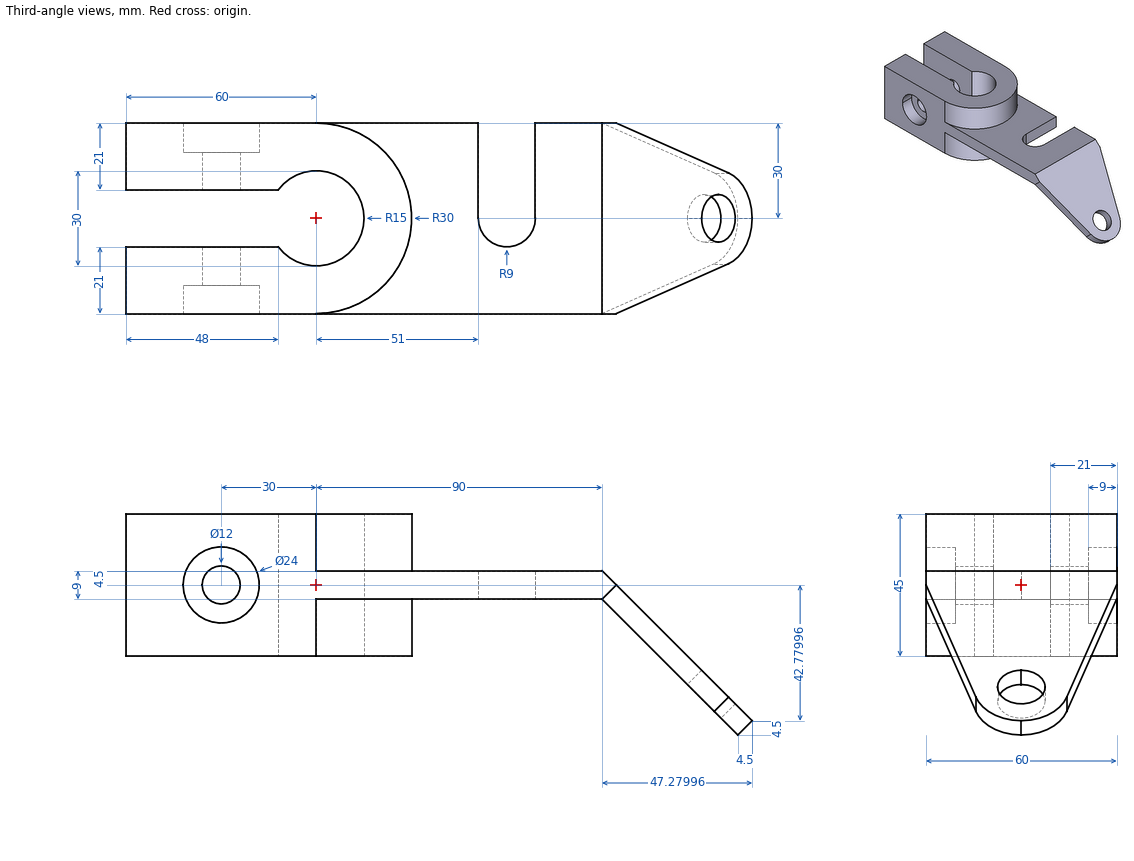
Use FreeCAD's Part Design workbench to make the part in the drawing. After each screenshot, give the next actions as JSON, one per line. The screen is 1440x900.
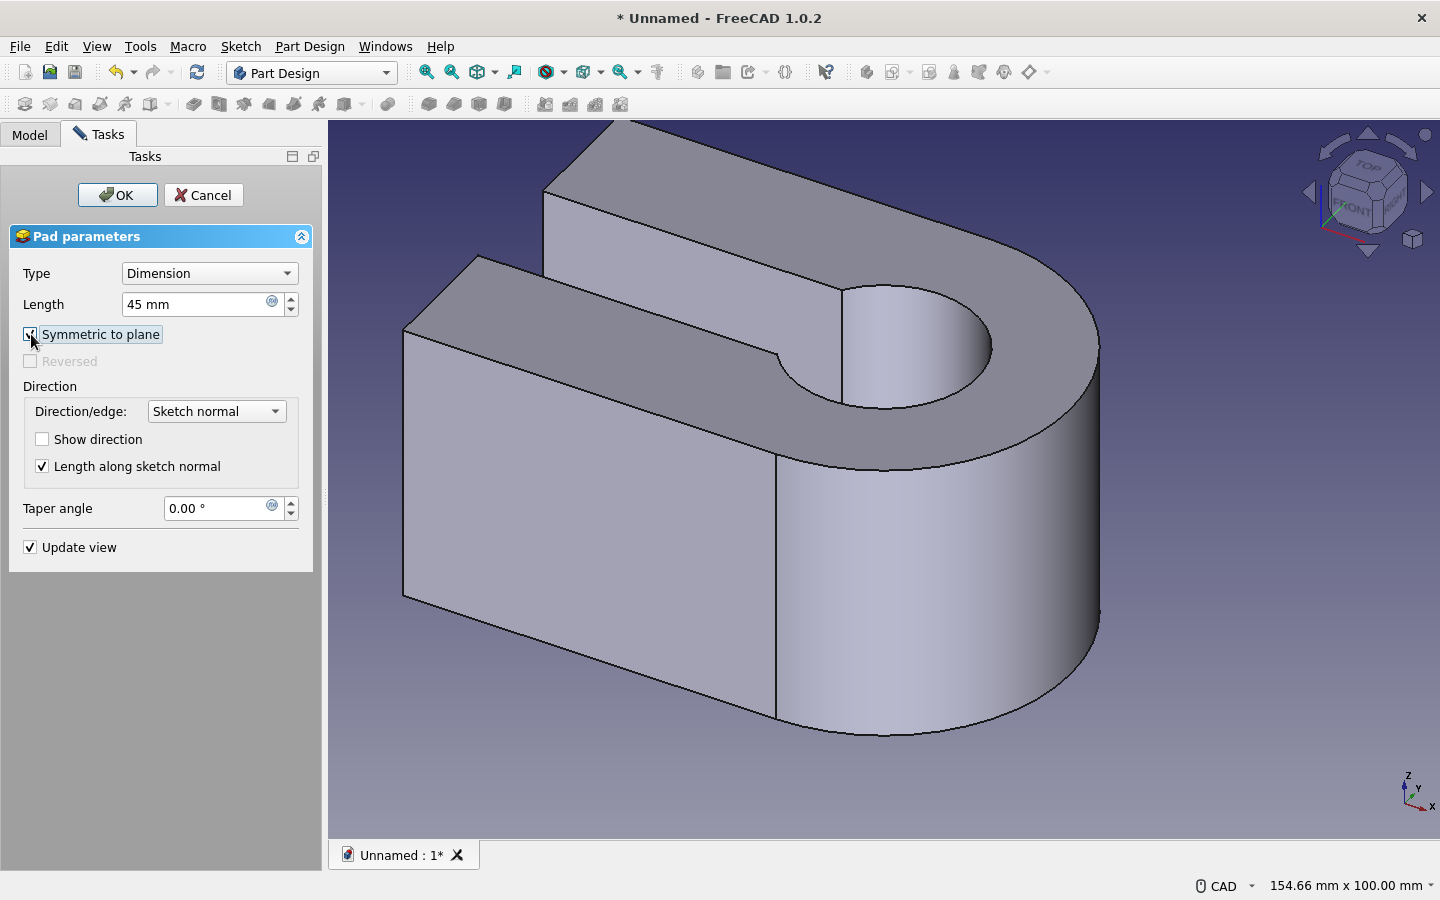
{"action": "left_click", "coordinate": [118, 195]}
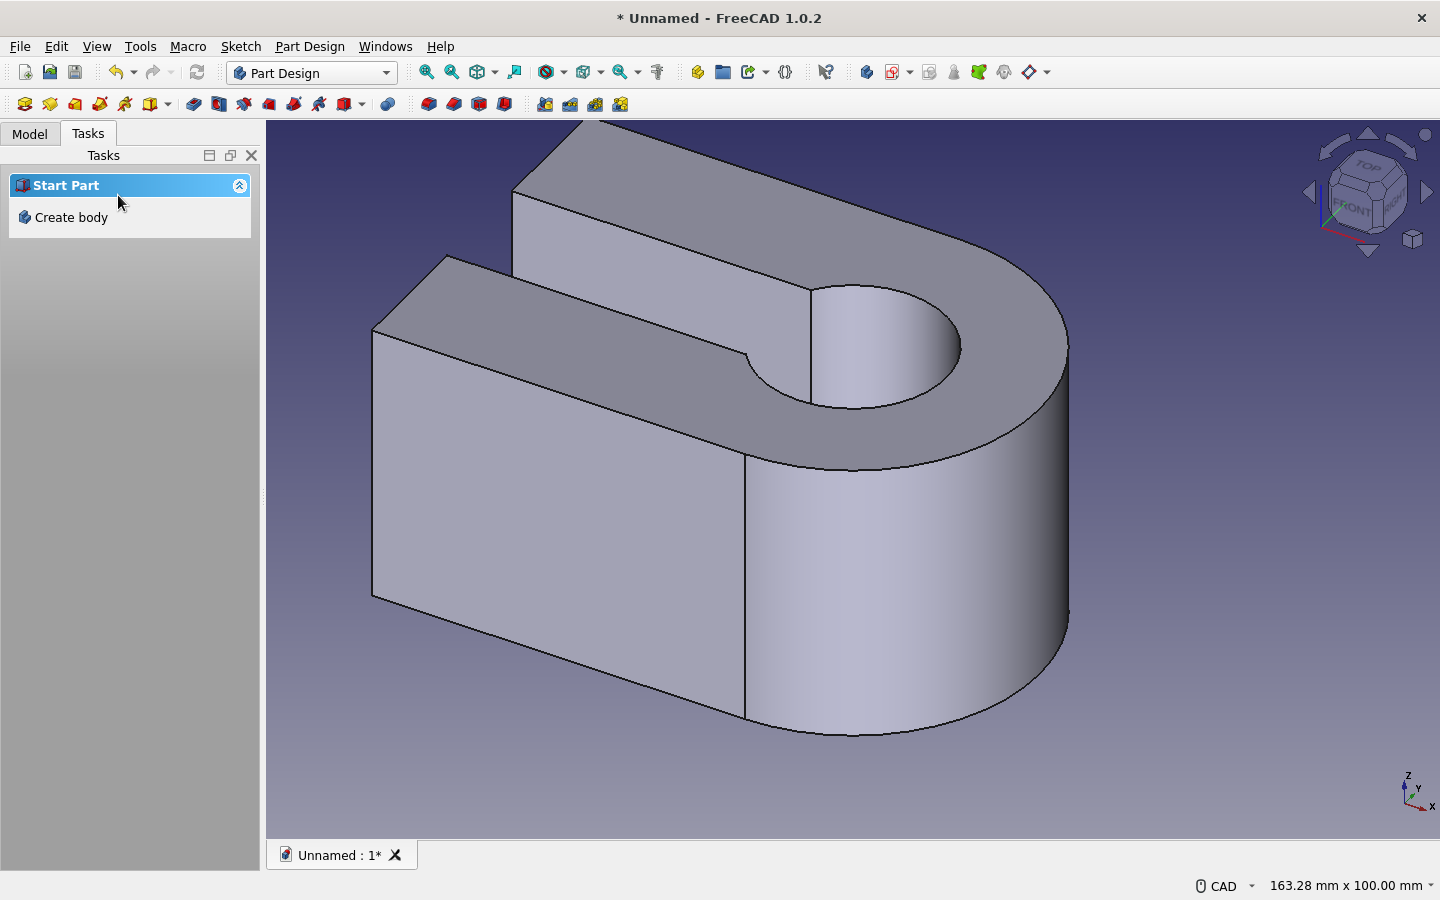
{"action": "left_click", "coordinate": [427, 72]}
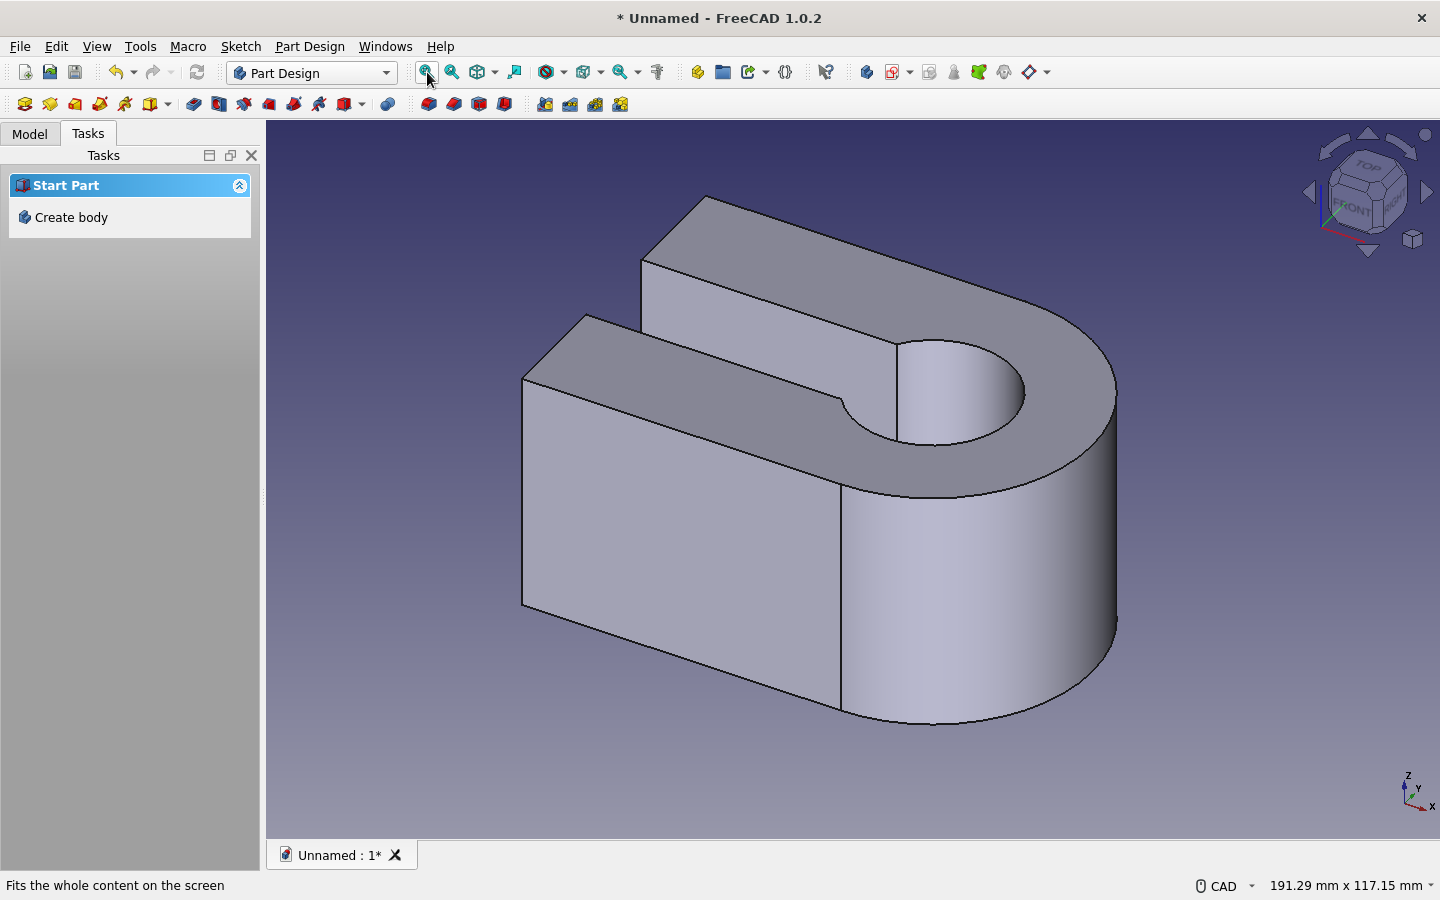
{"action": "key", "text": "4"}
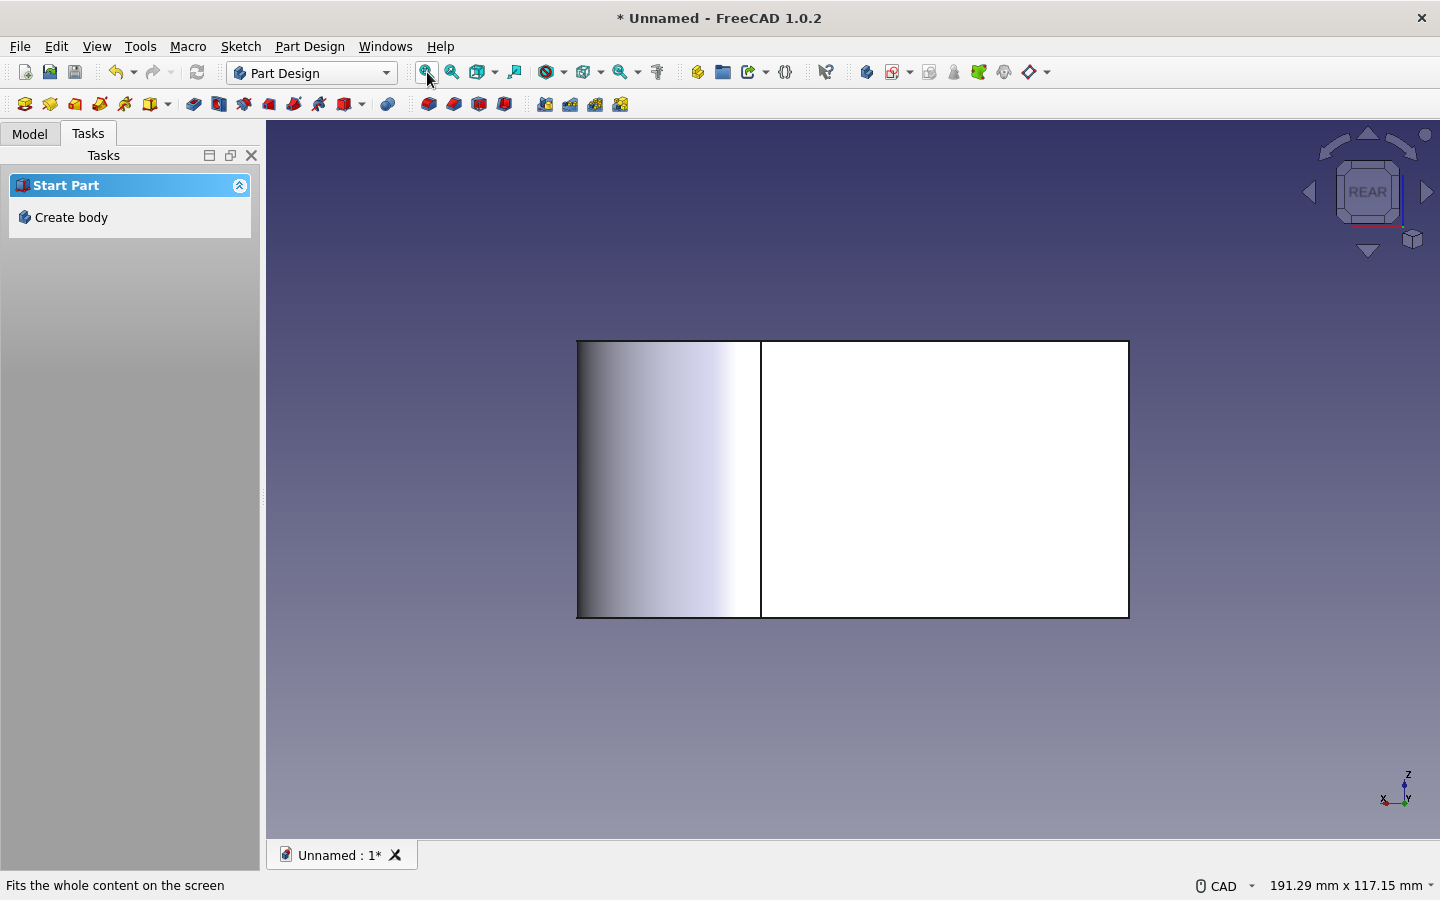
{"action": "left_click", "coordinate": [945, 478]}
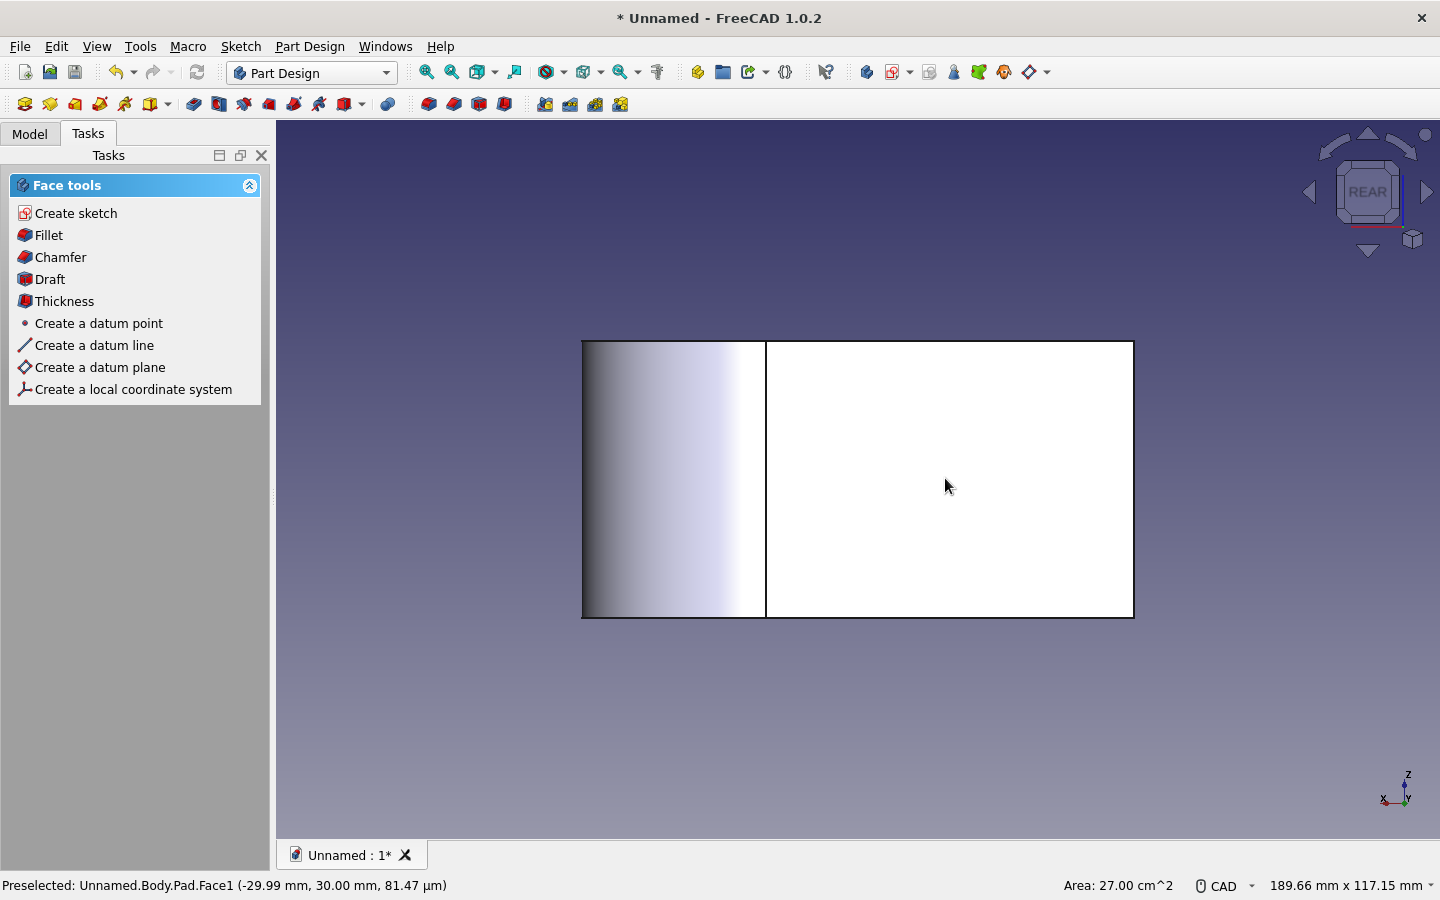
{"action": "left_click", "coordinate": [892, 72]}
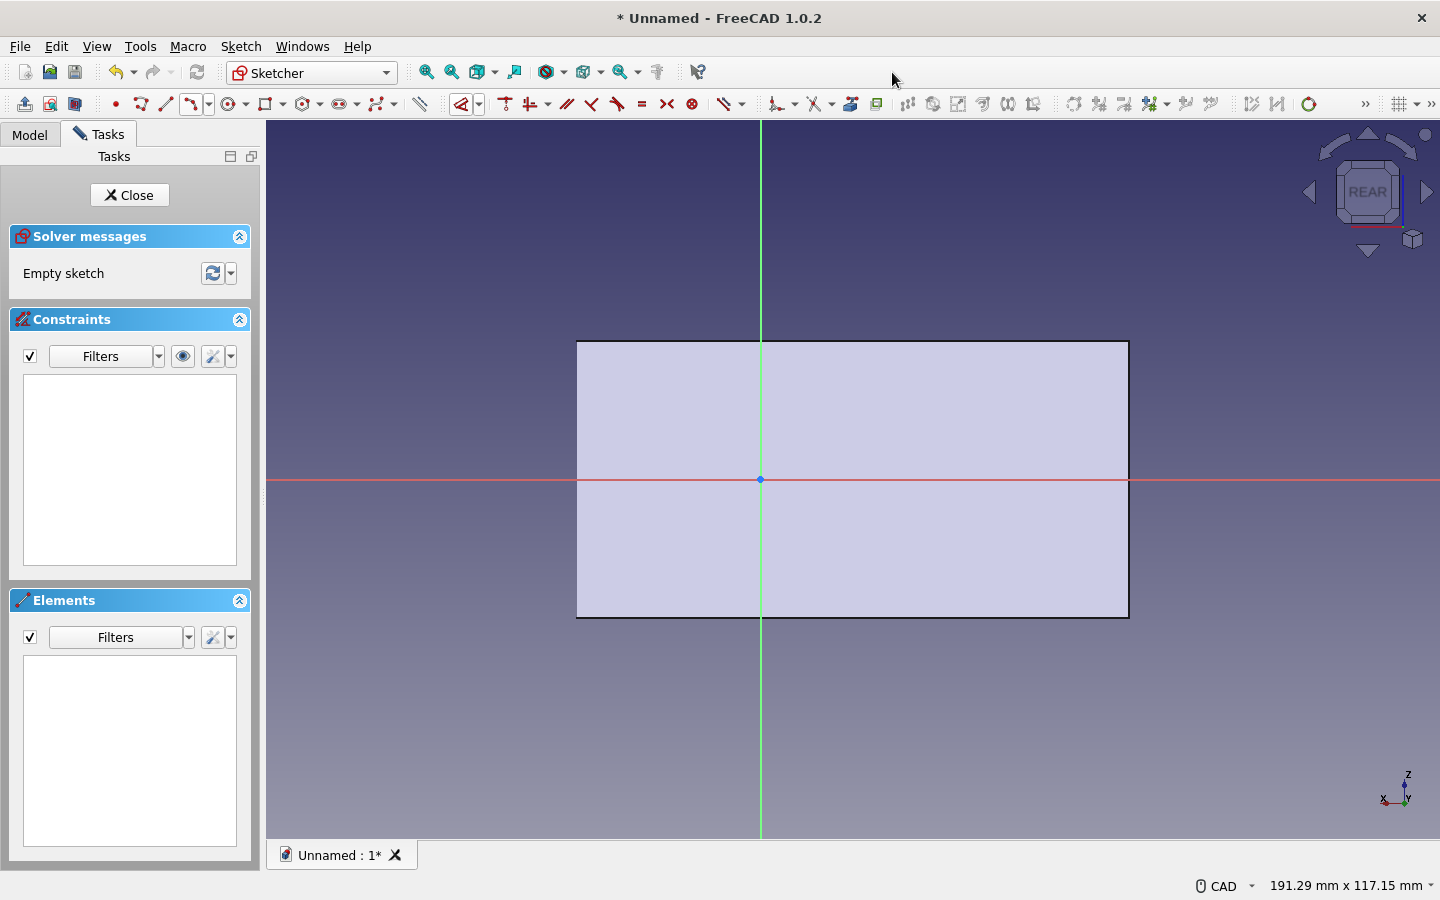
{"action": "scroll", "coordinate": [951, 479], "scroll_direction": "up", "scroll_amount": 5}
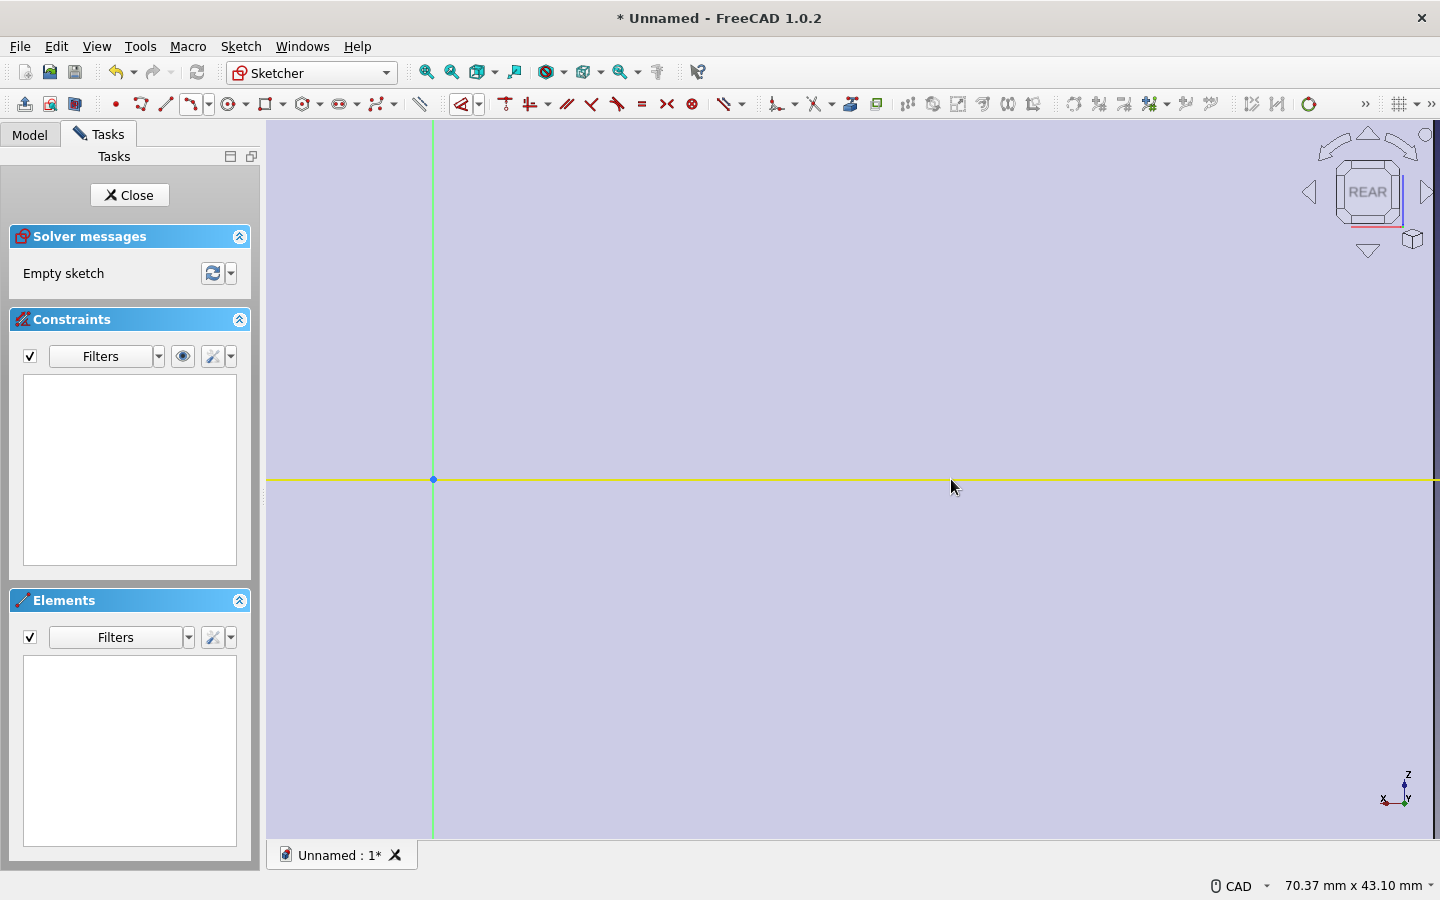
{"action": "left_click", "coordinate": [228, 104]}